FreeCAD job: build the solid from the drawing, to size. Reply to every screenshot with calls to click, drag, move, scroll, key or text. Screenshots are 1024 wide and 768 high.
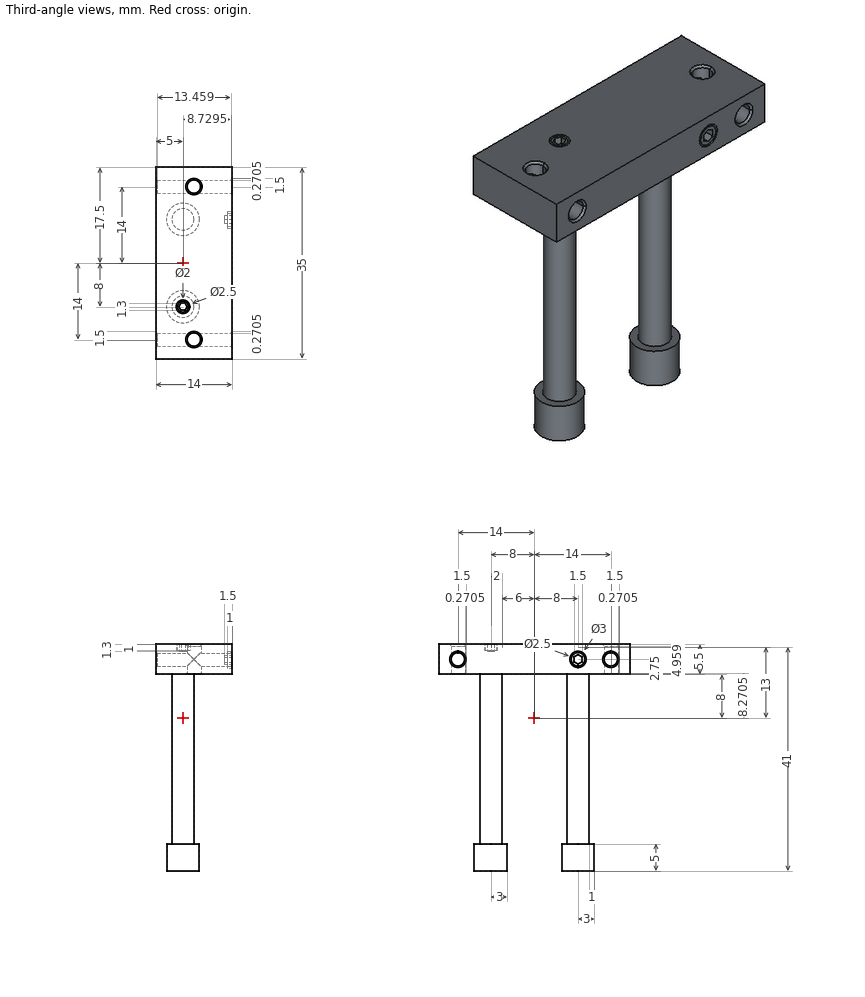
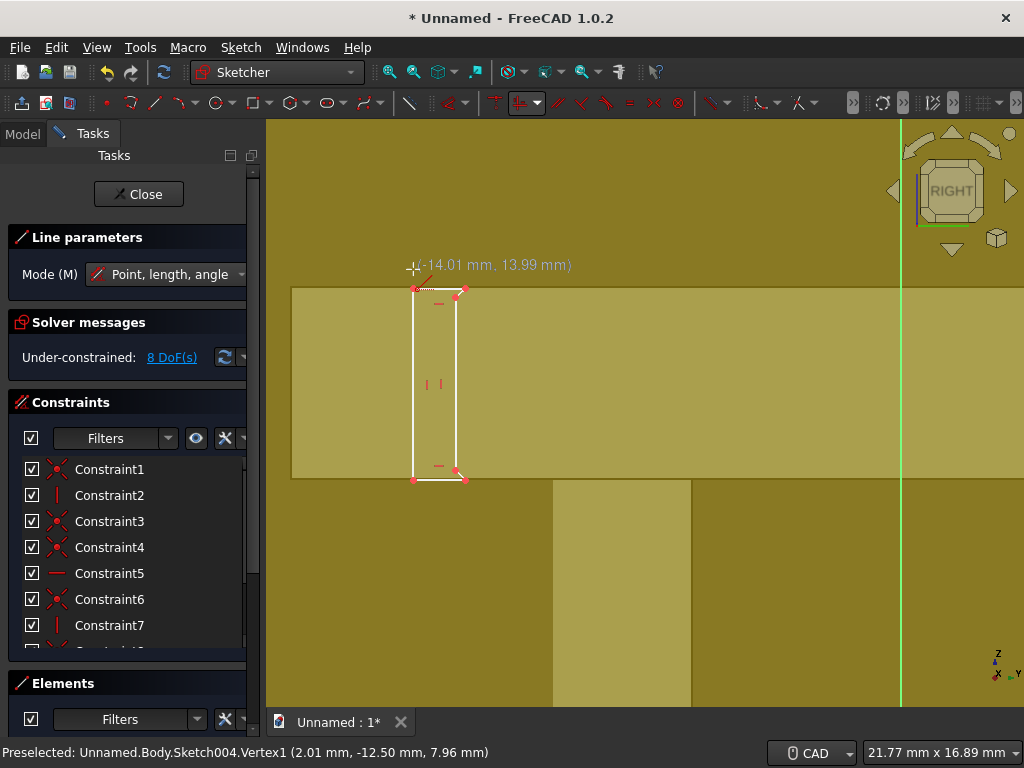
click(413, 268)
click(413, 211)
key(Escape)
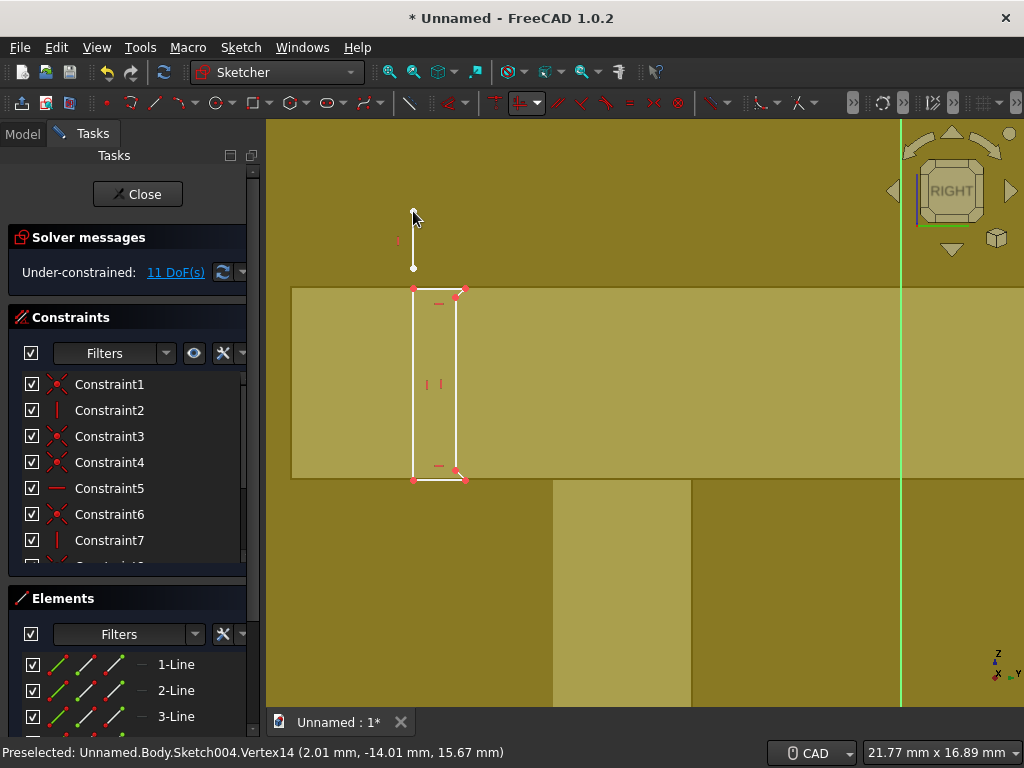
click(413, 252)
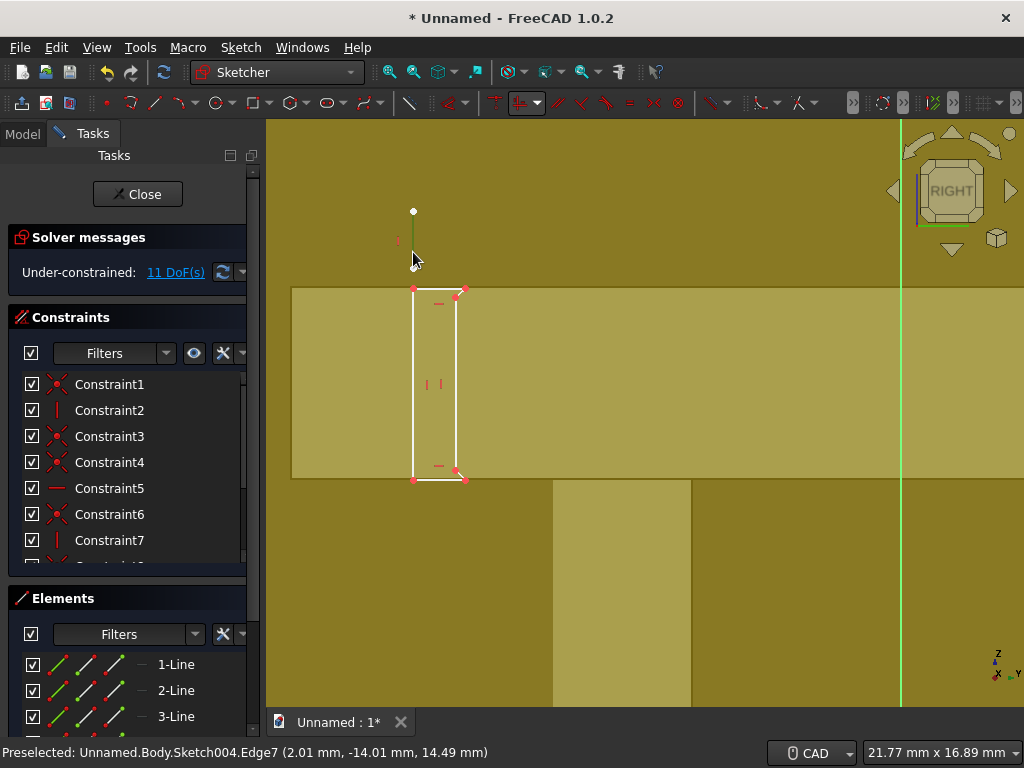
click(410, 104)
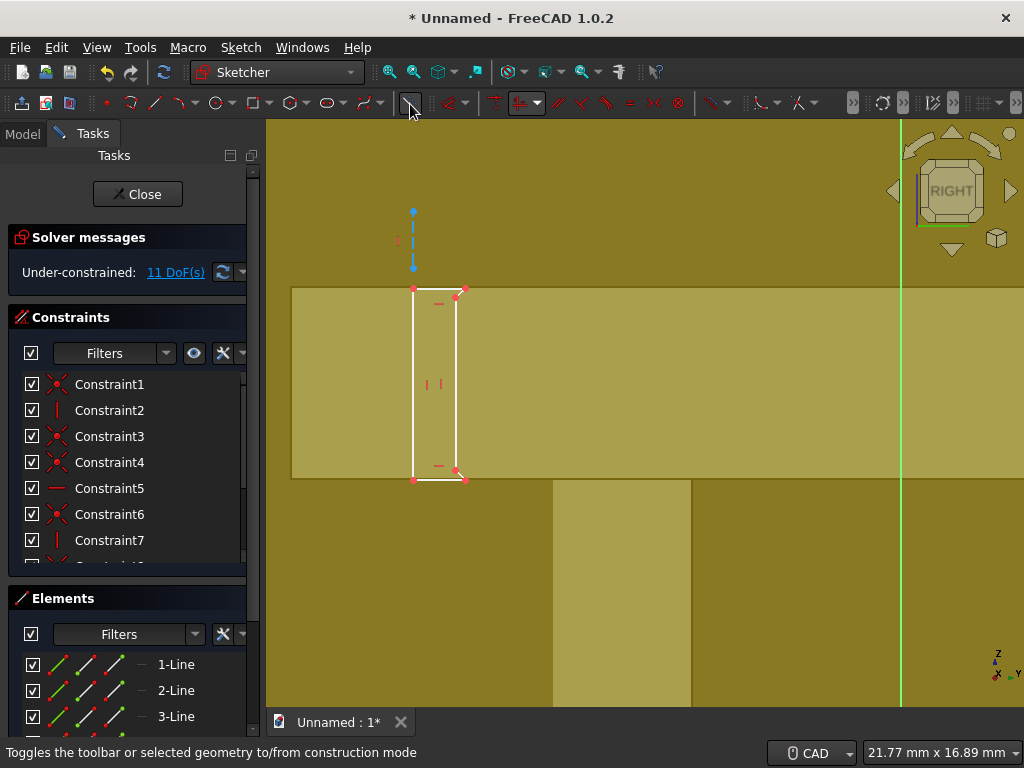
click(448, 104)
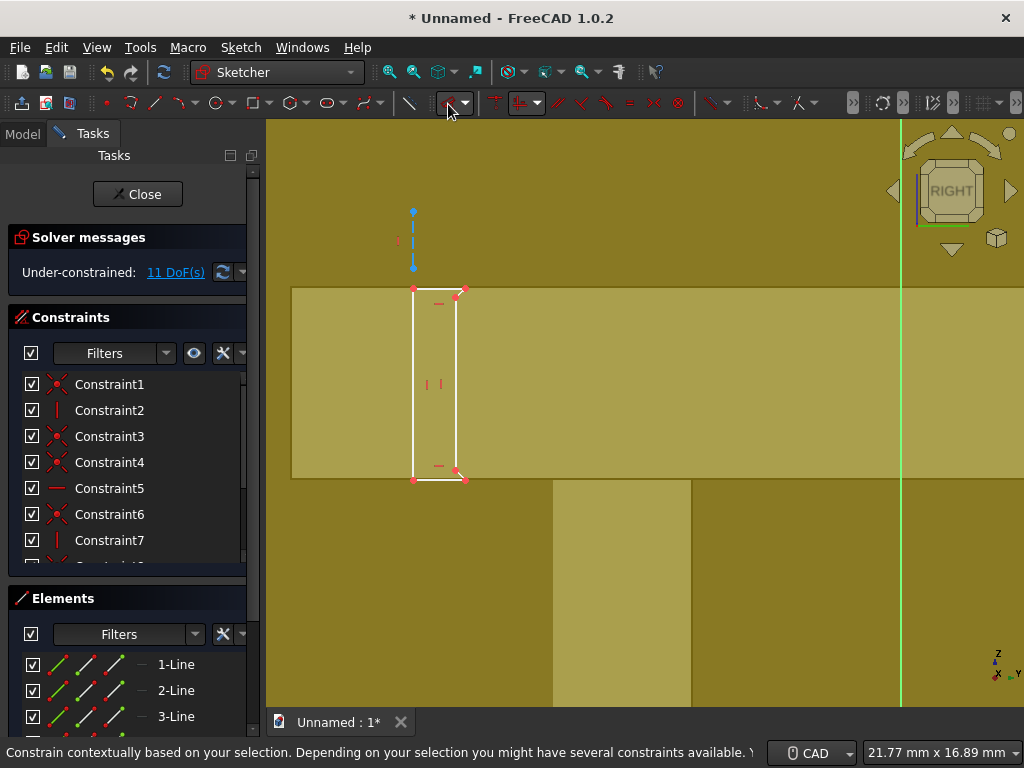
click(465, 480)
click(431, 580)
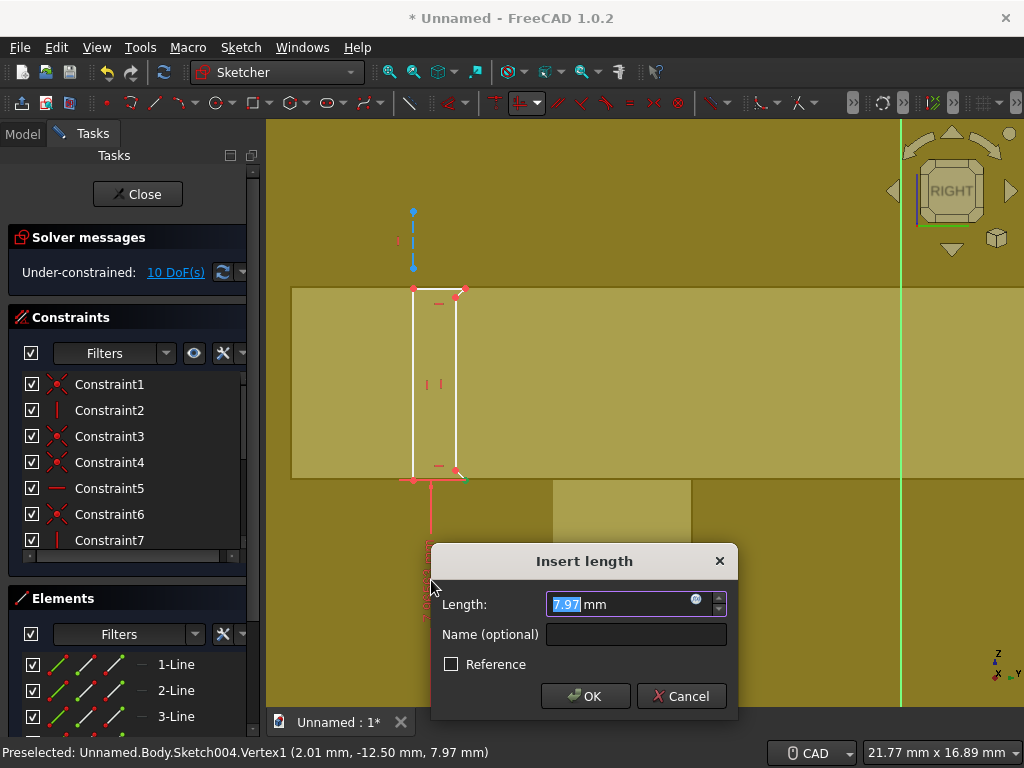
text(8)
key(Return)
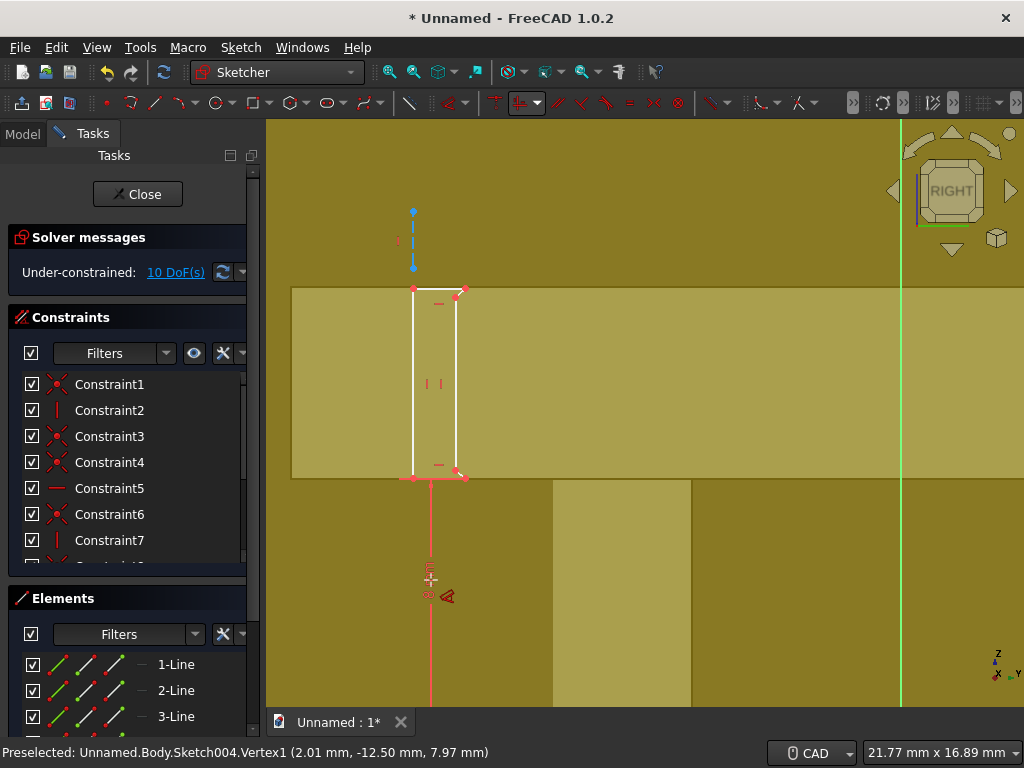
scroll(450, 289, up, 2)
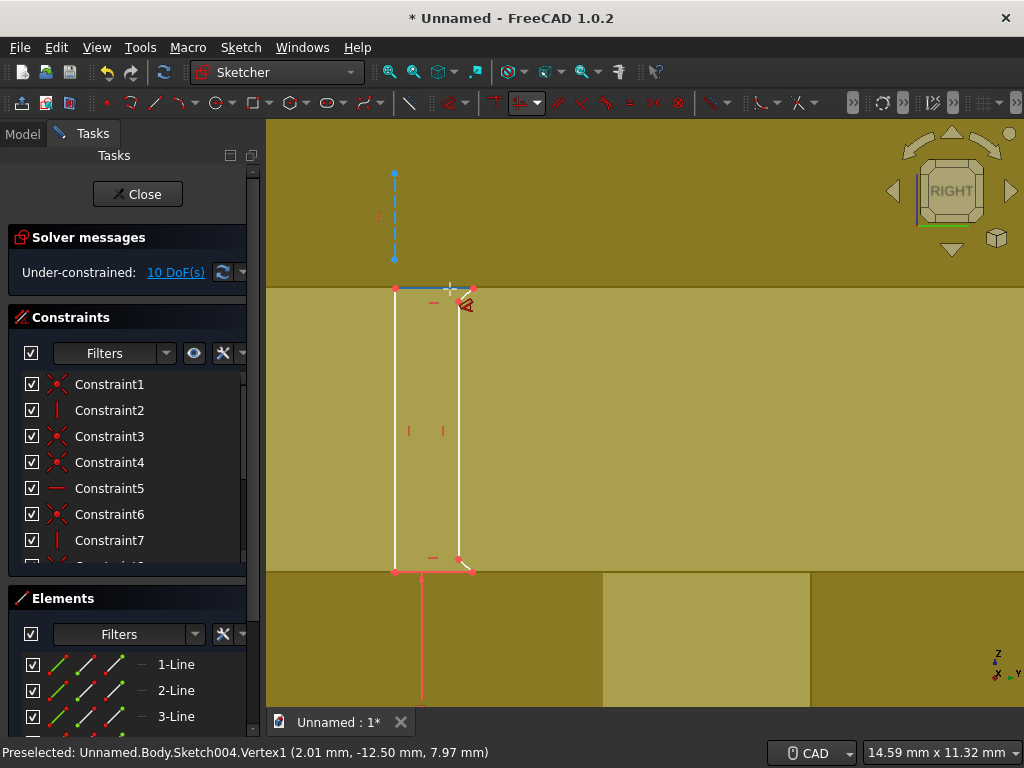
click(450, 288)
click(434, 254)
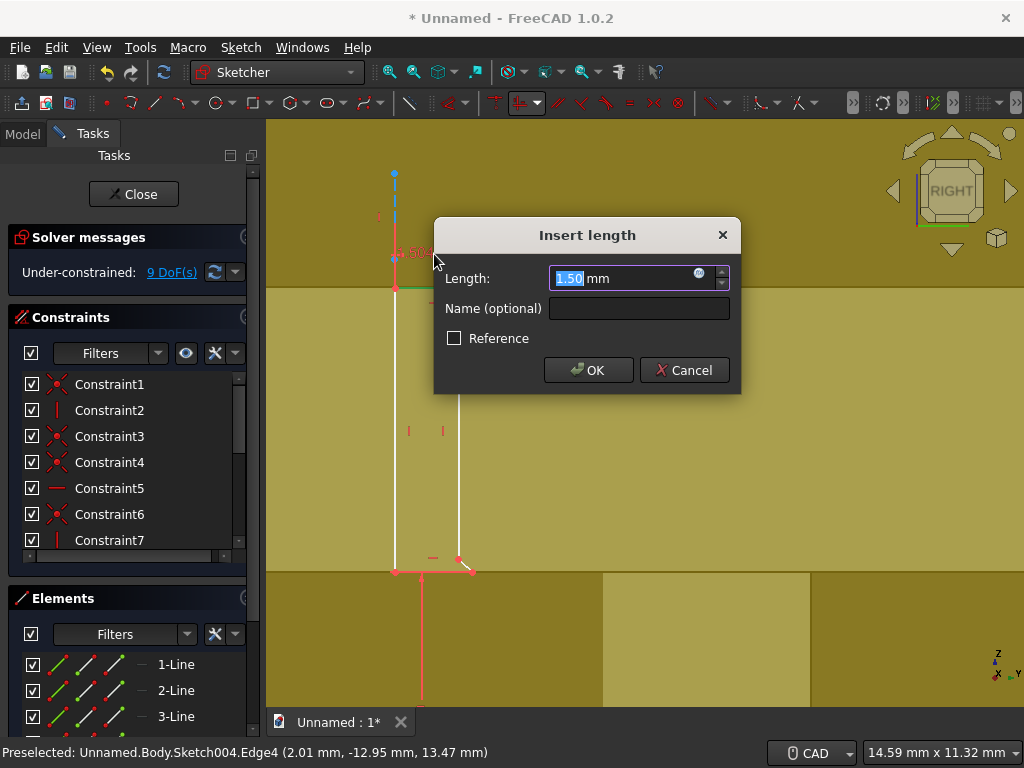
text(1.5)
key(Return)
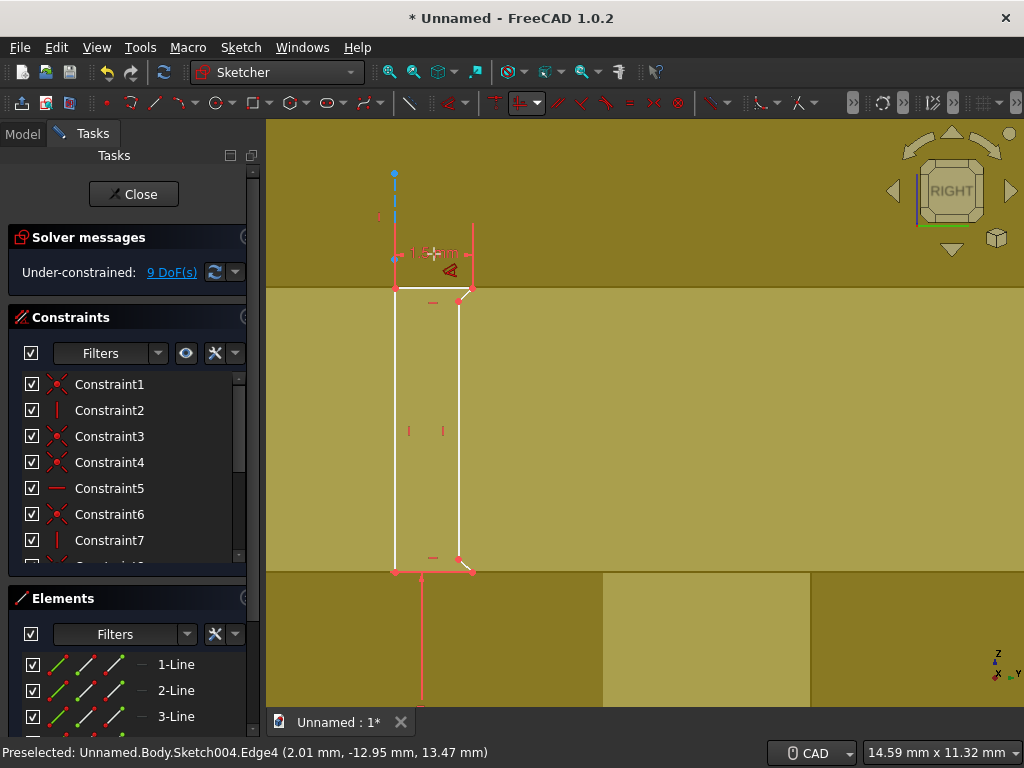
click(395, 373)
click(361, 430)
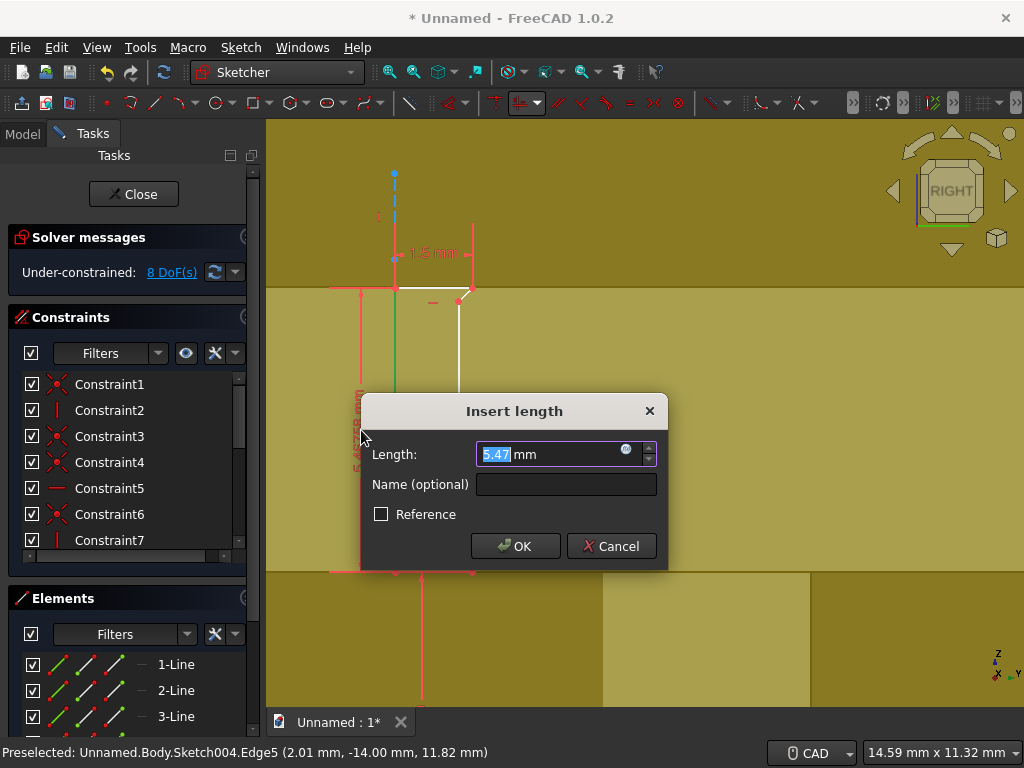
text(5.5)
key(Return)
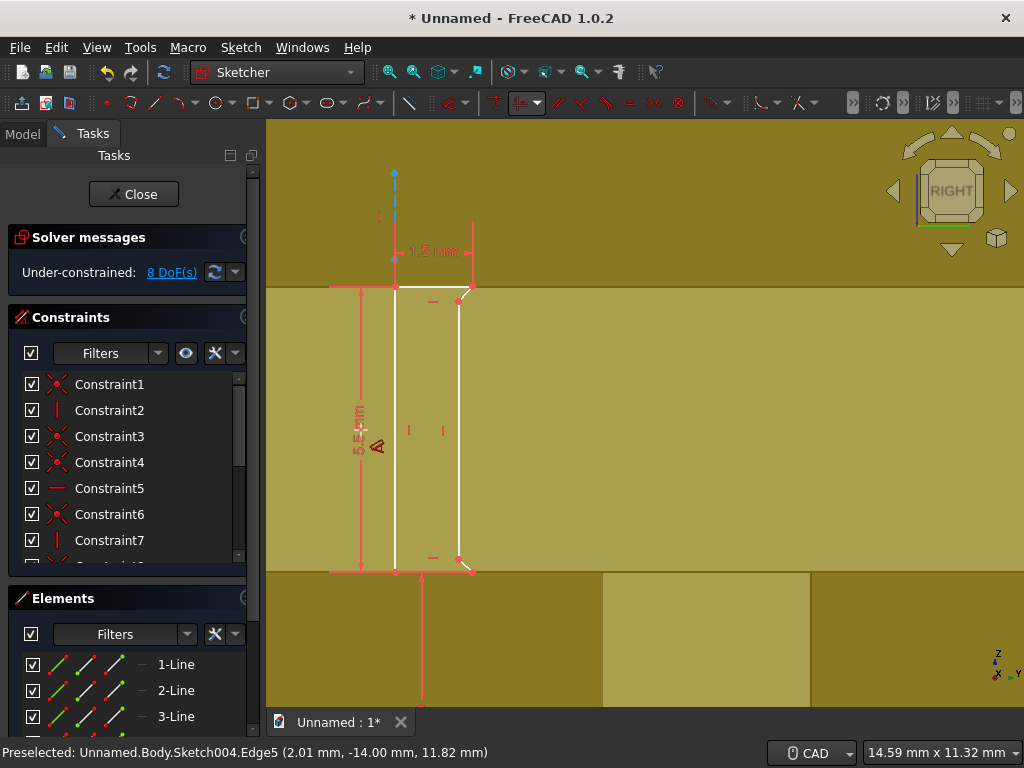
click(418, 572)
click(434, 538)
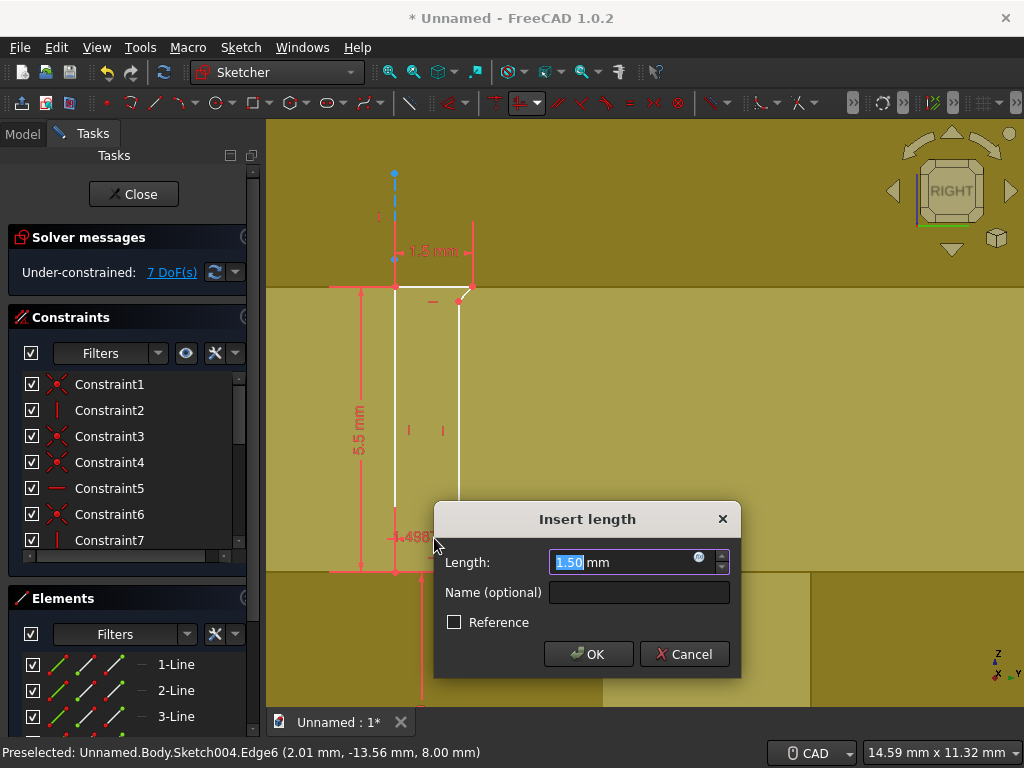
text(1.5)
key(Return)